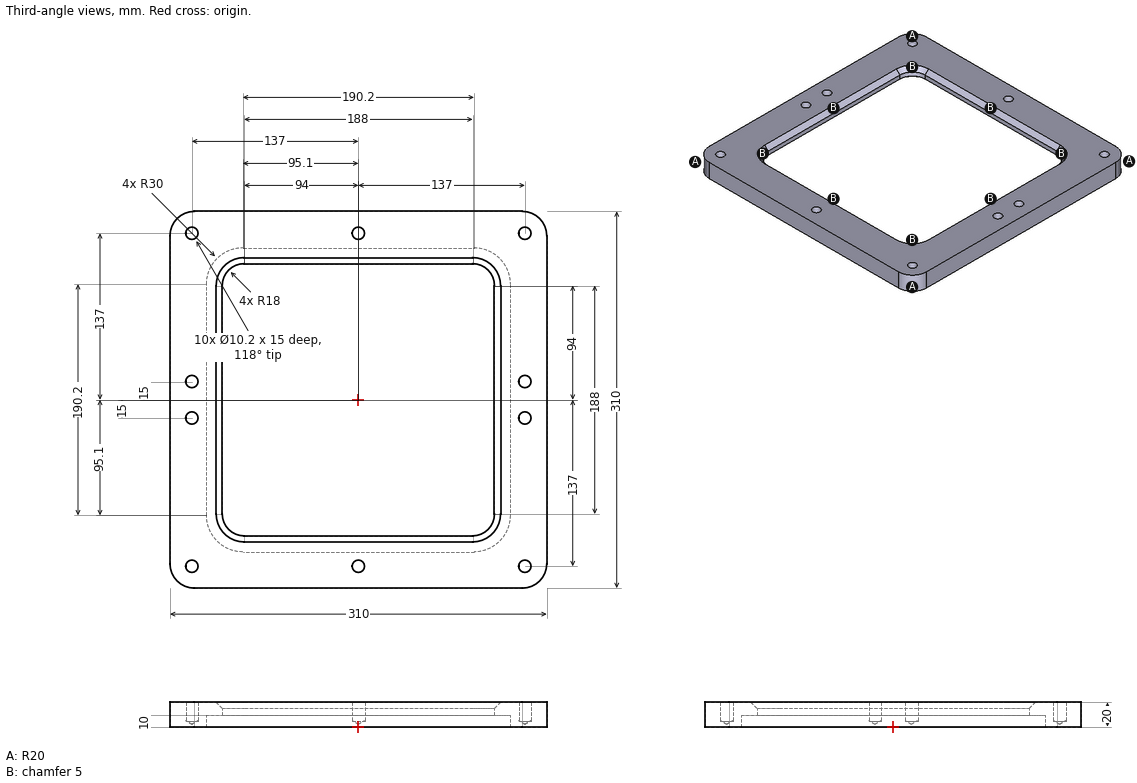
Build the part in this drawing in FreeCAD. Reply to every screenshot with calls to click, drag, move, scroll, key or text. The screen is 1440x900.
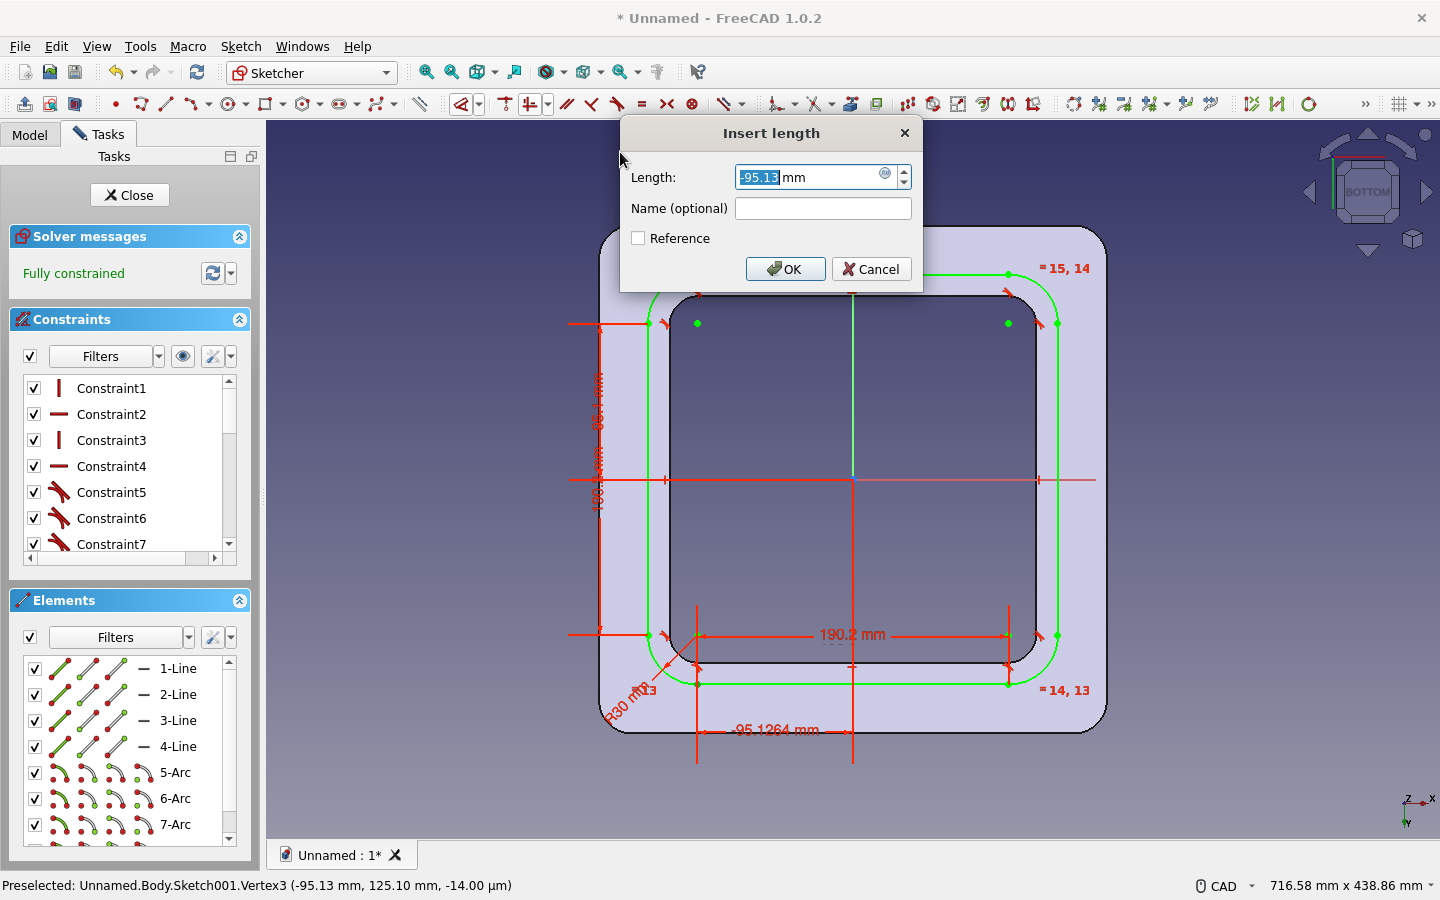
text(-95.1)
key(Return)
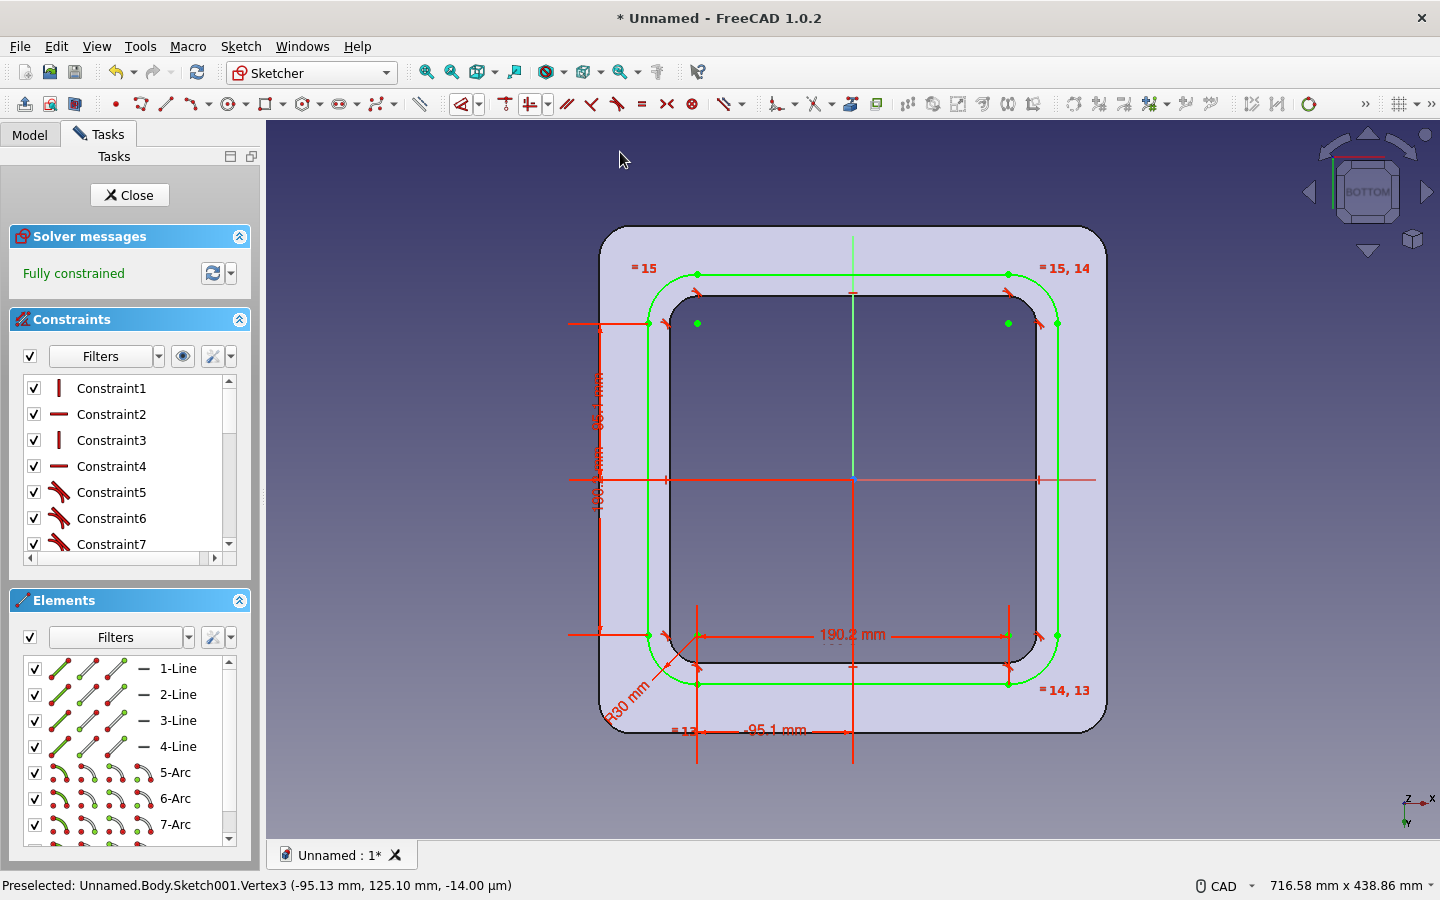
click(130, 195)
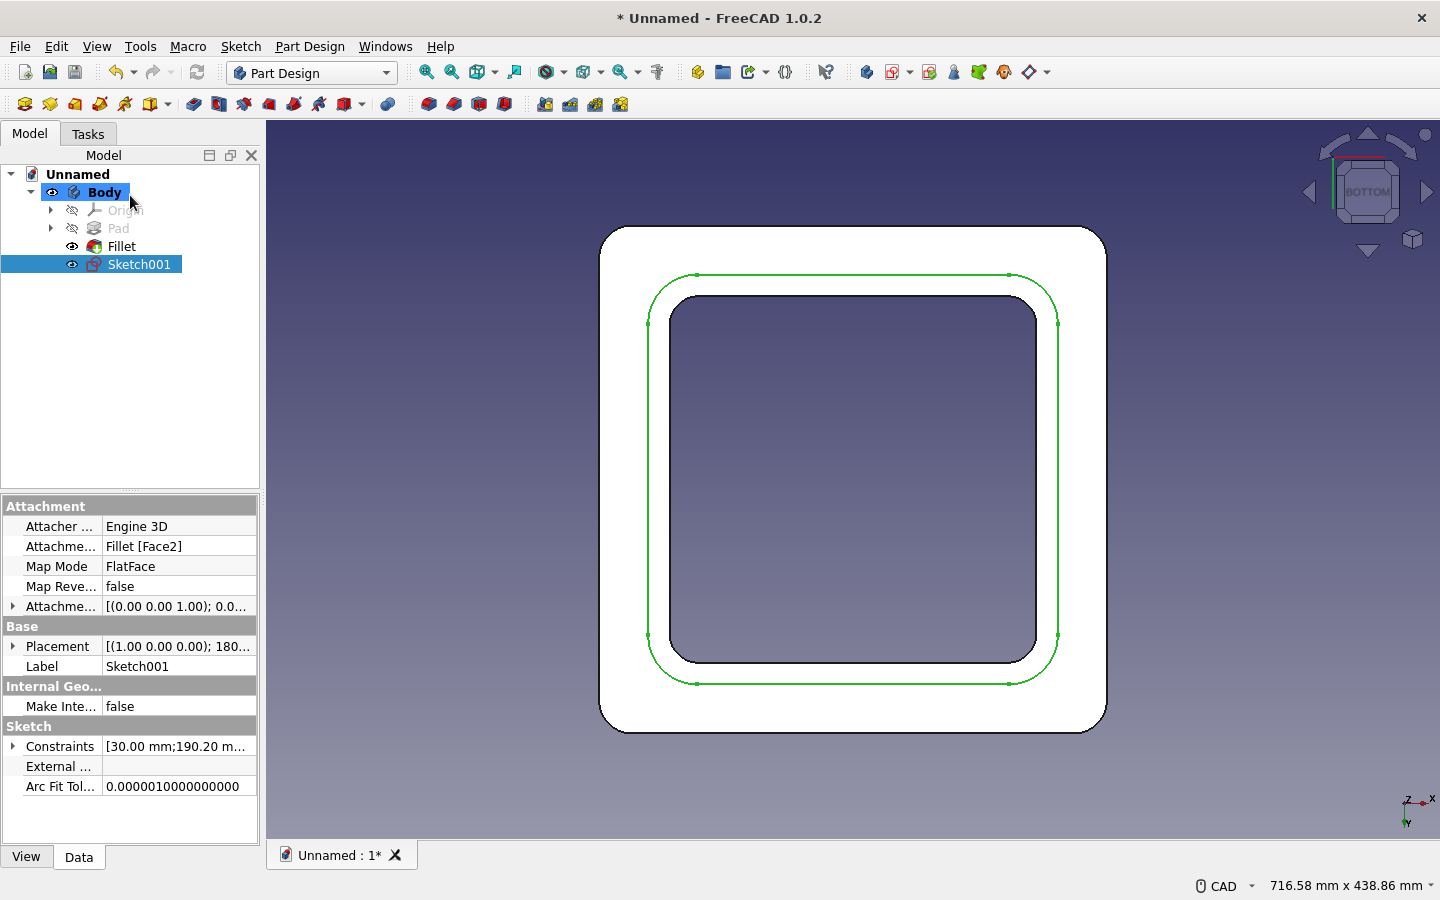
click(194, 104)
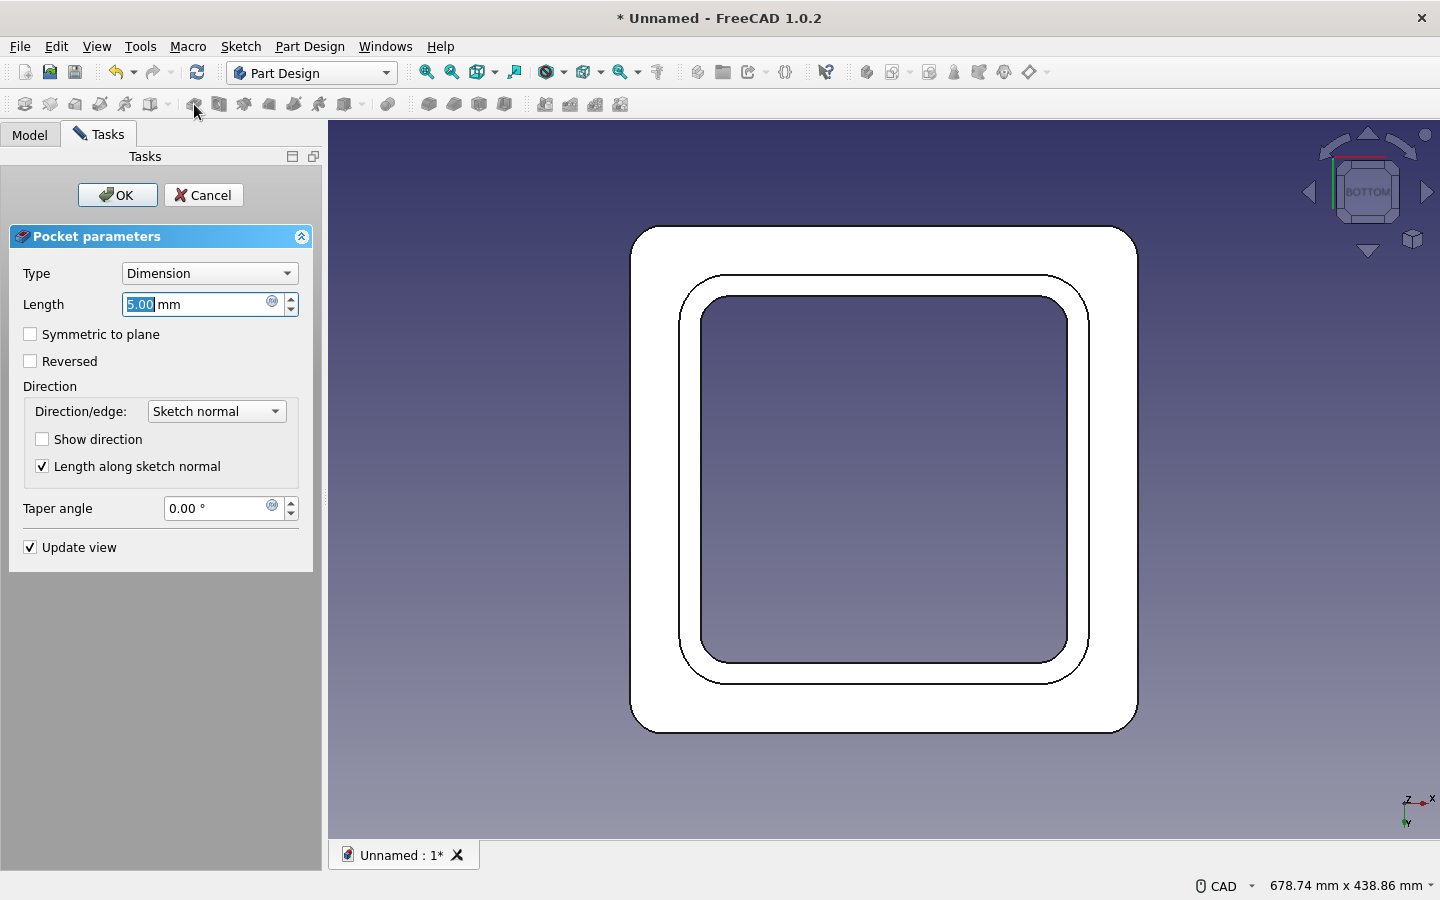
text(10)
key(Tab)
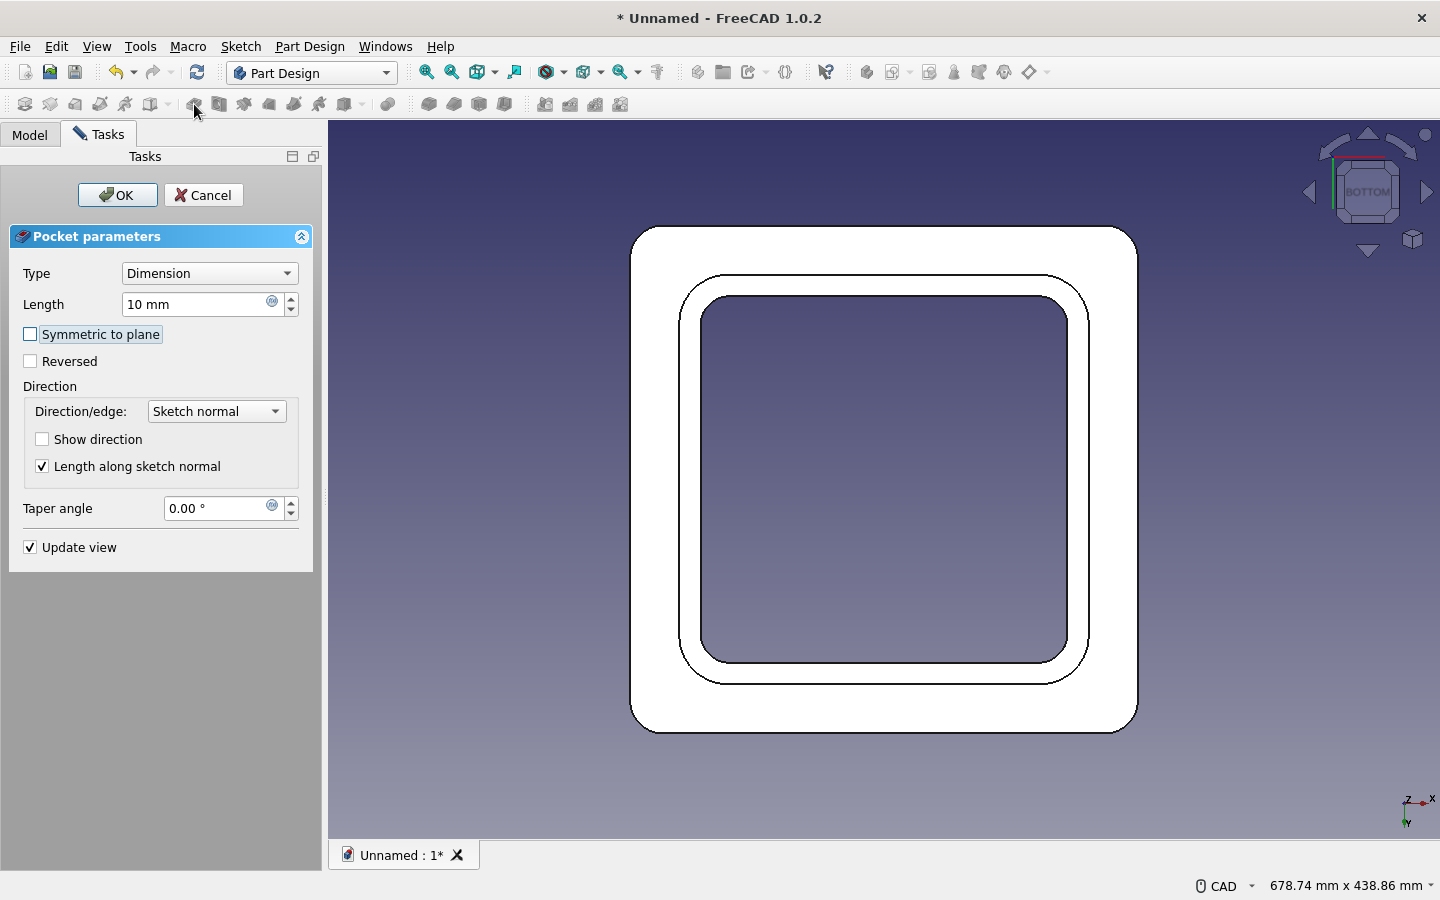
click(118, 195)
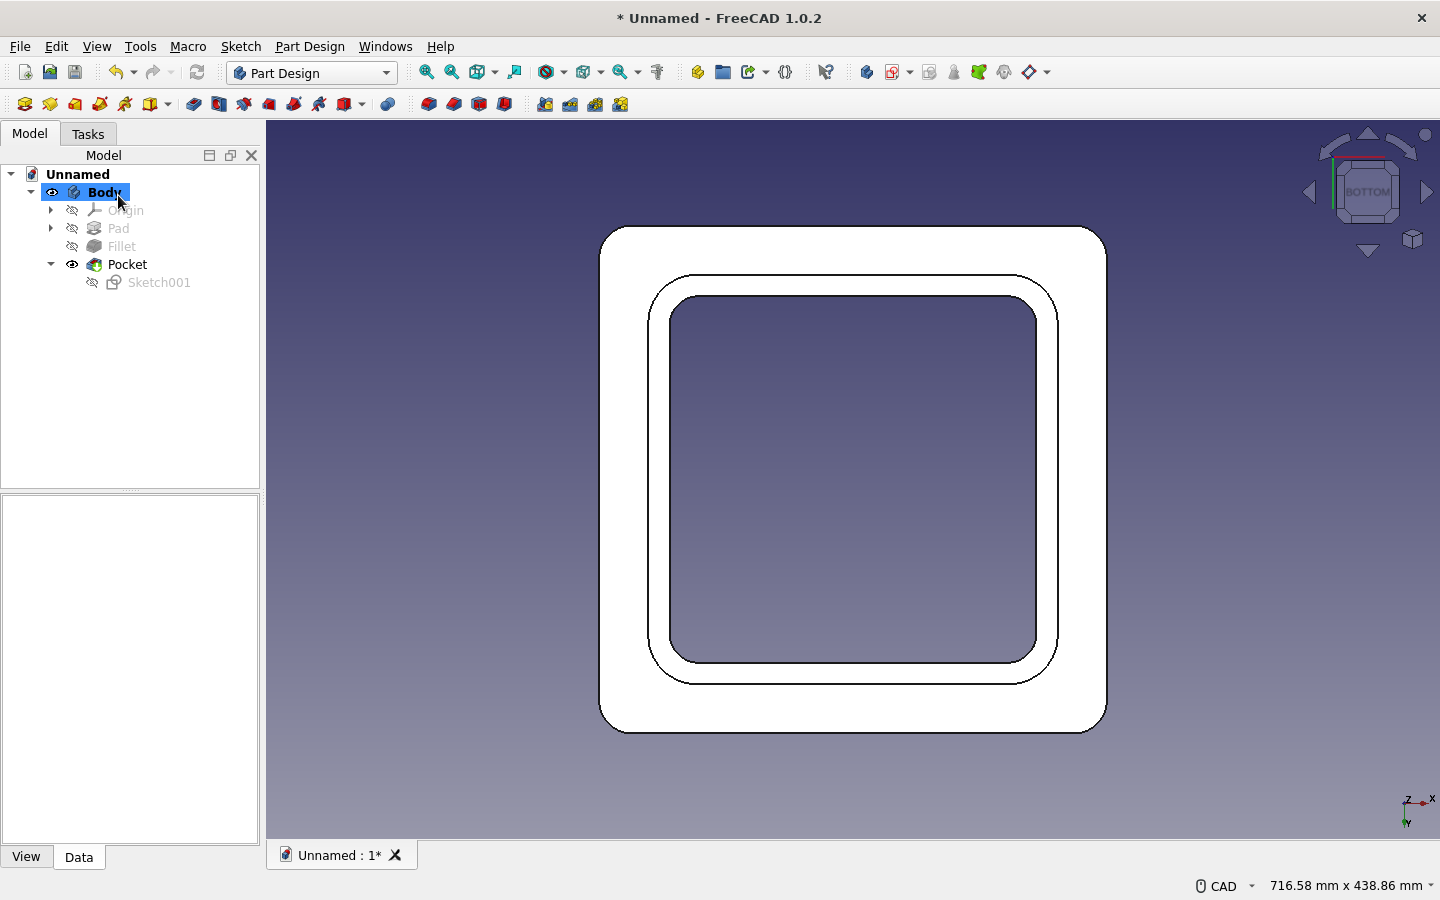
key(0)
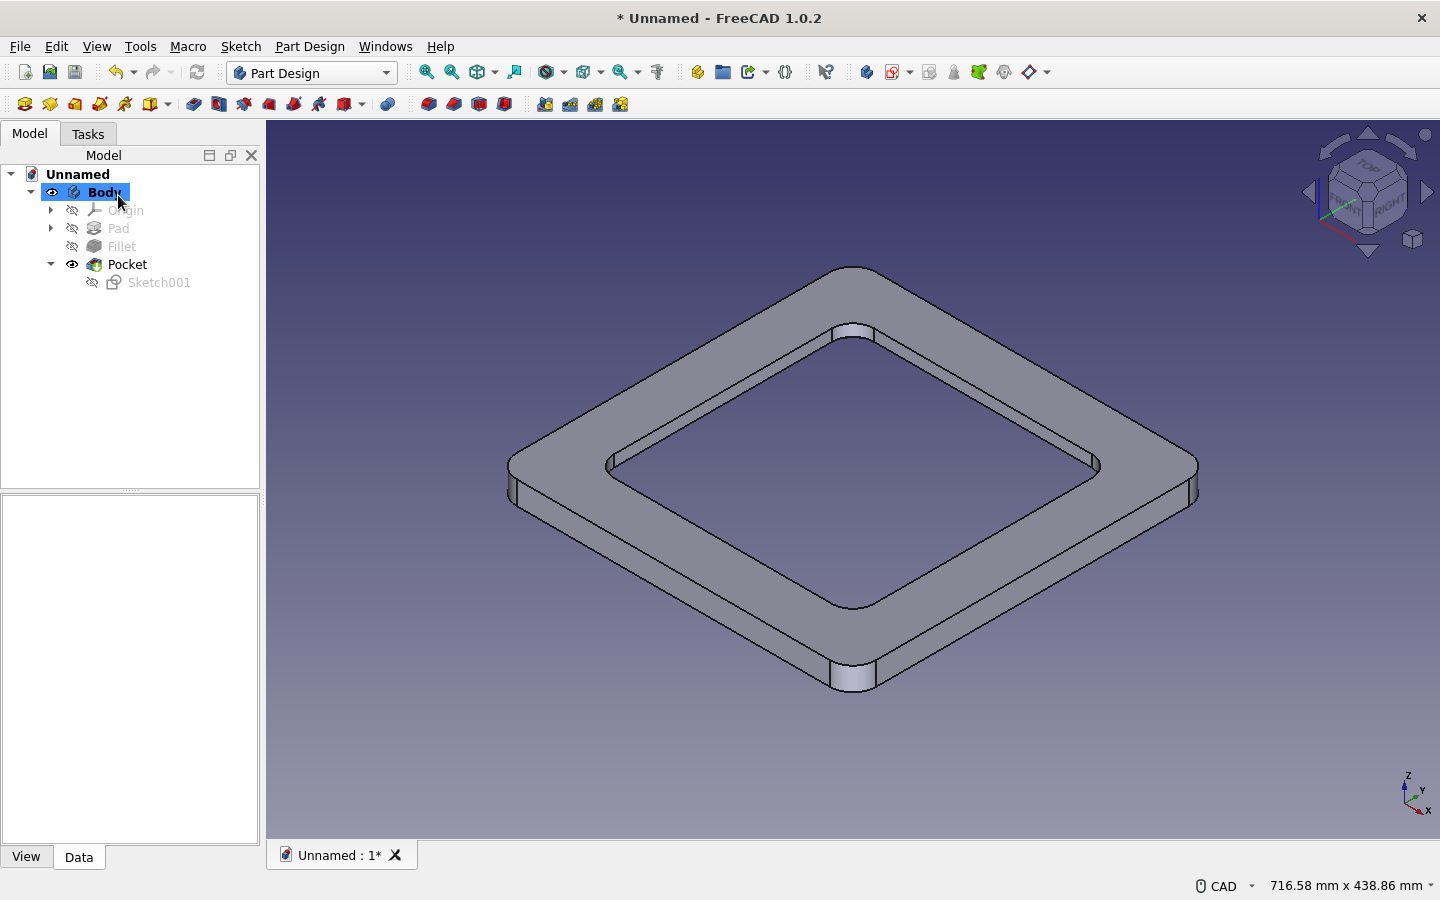
click(1161, 465)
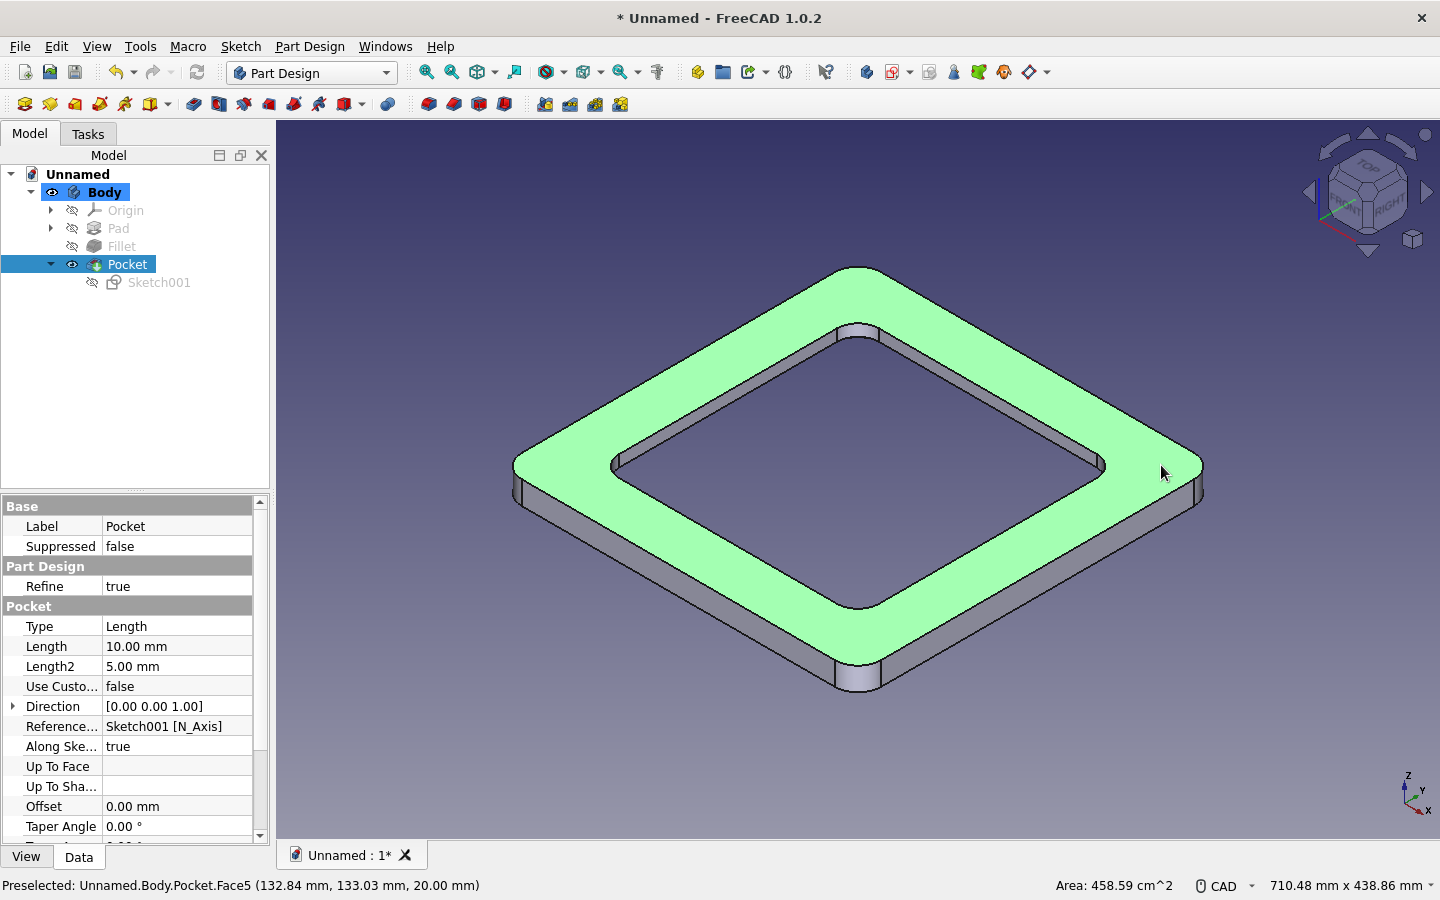
click(892, 72)